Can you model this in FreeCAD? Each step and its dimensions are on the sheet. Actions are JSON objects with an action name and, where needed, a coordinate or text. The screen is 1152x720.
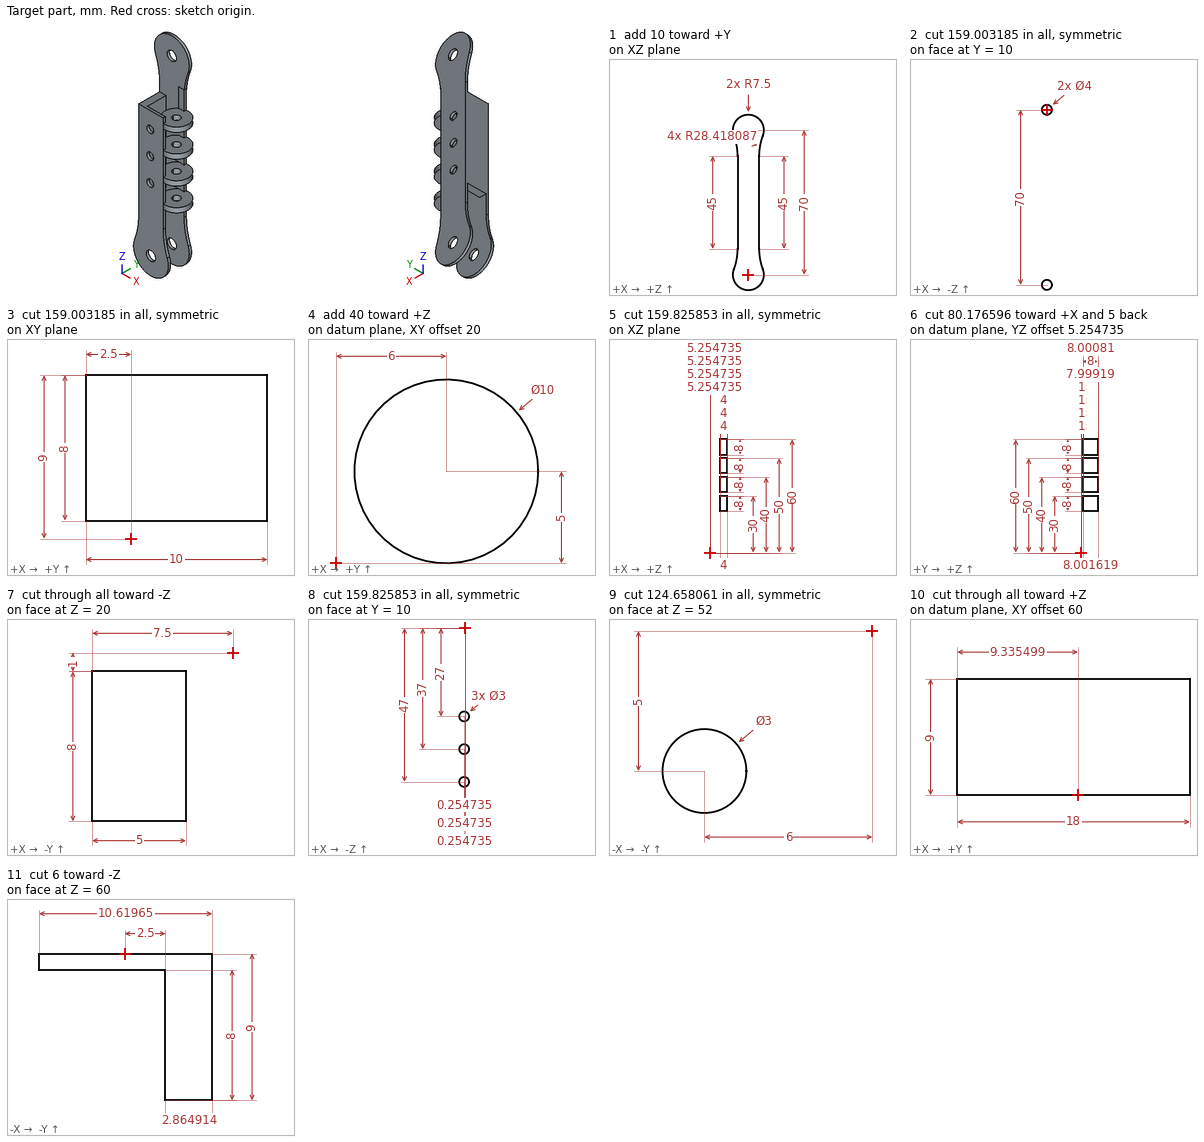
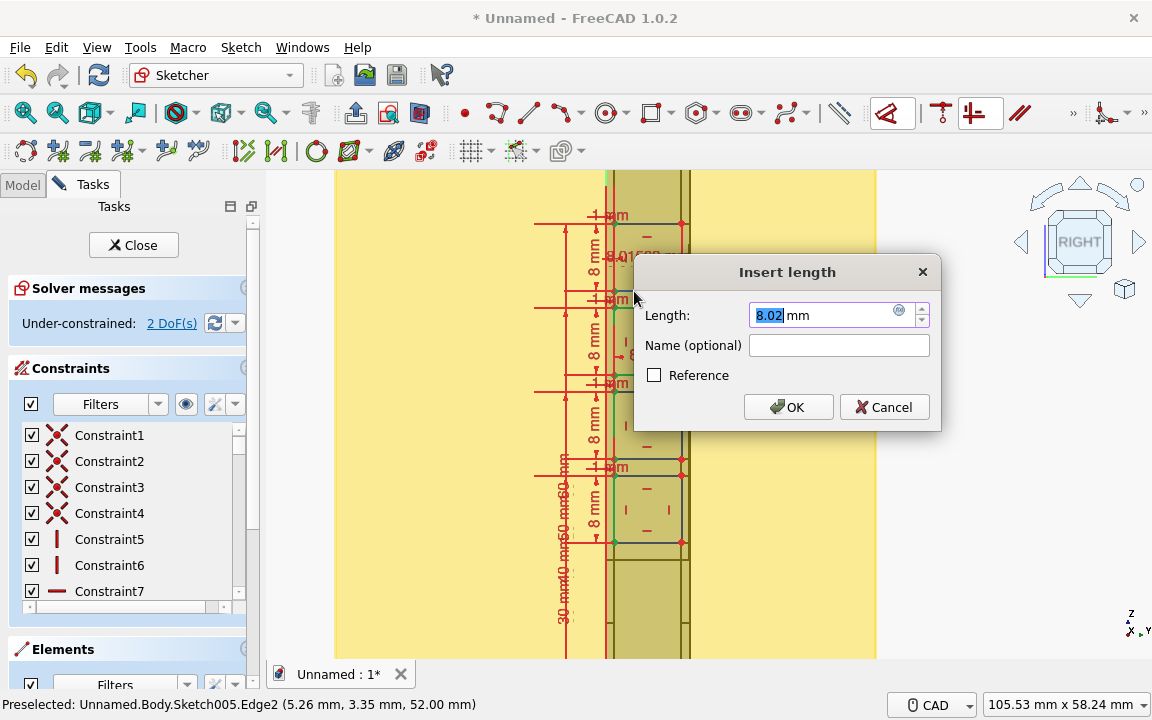
{"action": "type", "text": "7.99919"}
{"action": "key", "text": "Return"}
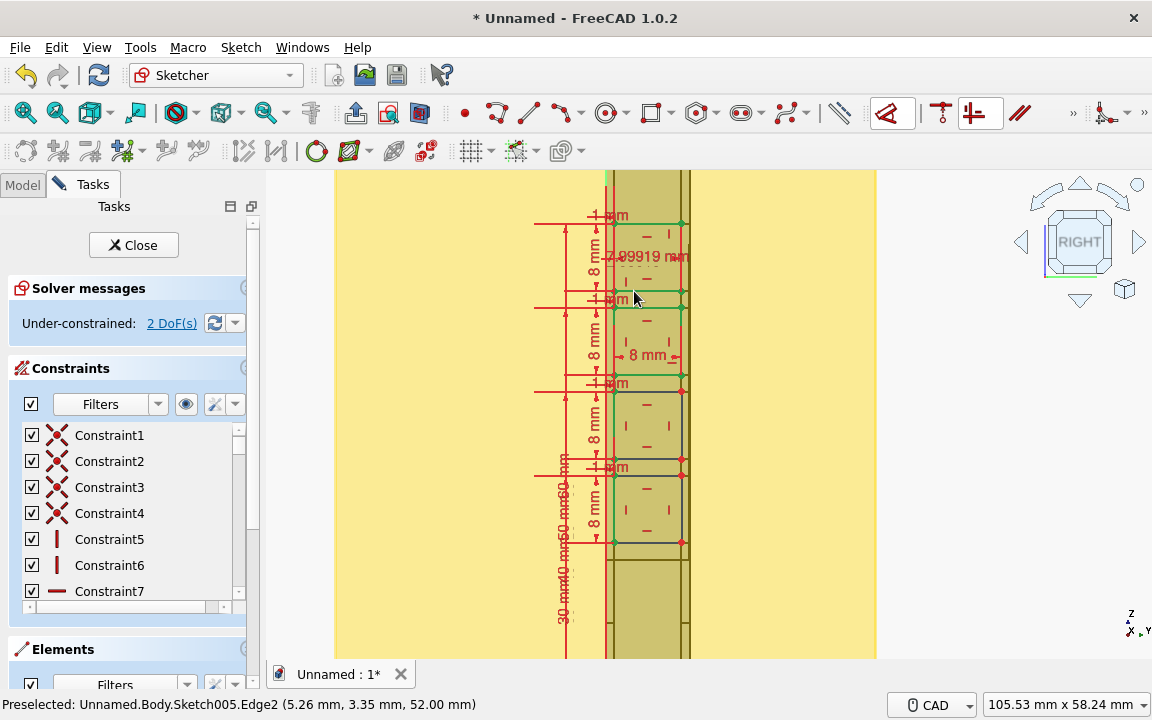
{"action": "left_click", "coordinate": [634, 459]}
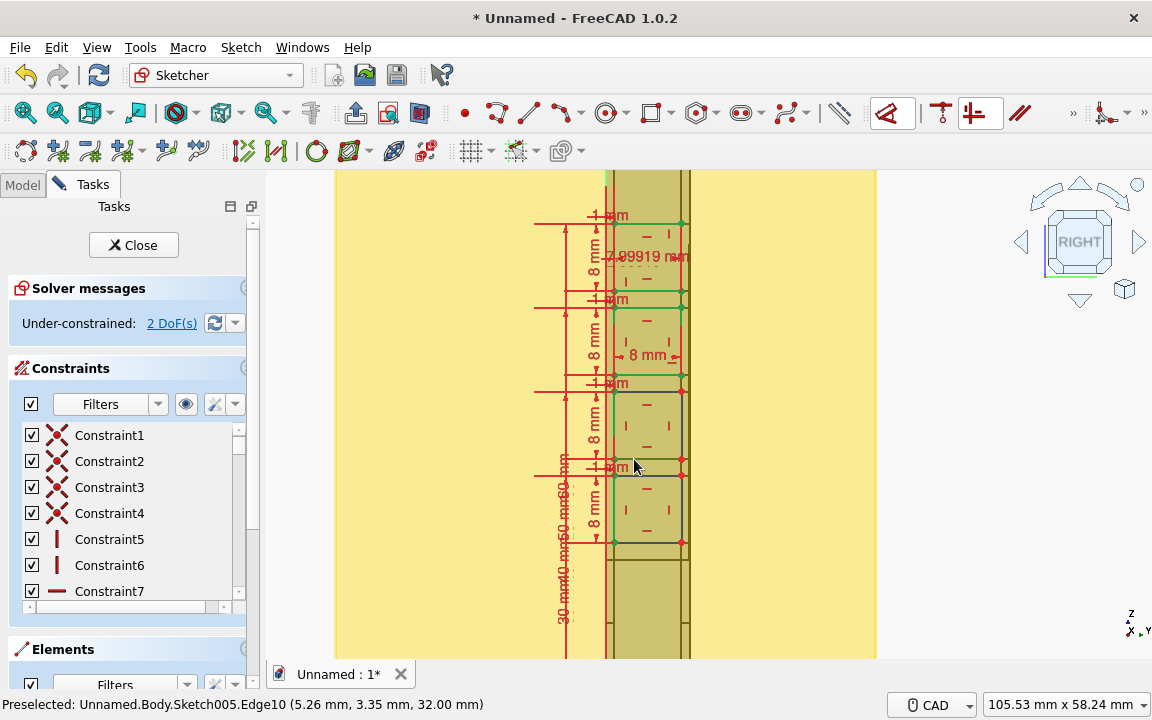
{"action": "key", "text": "l"}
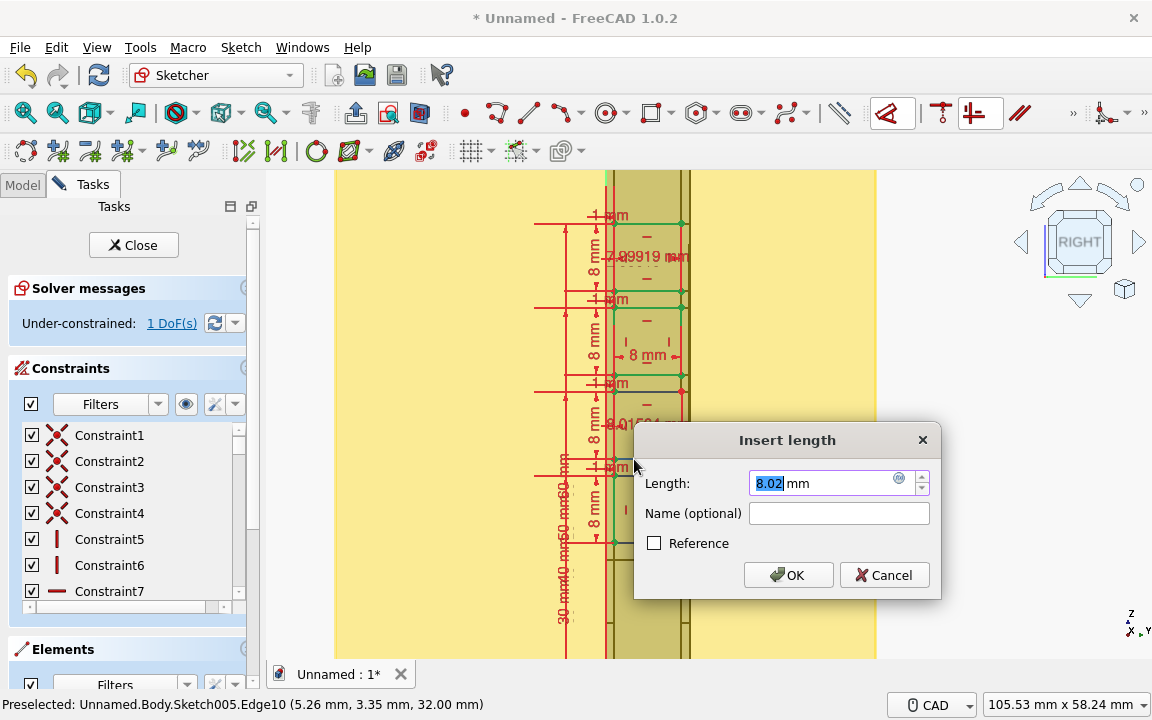
{"action": "type", "text": "8.00081"}
{"action": "key", "text": "Return"}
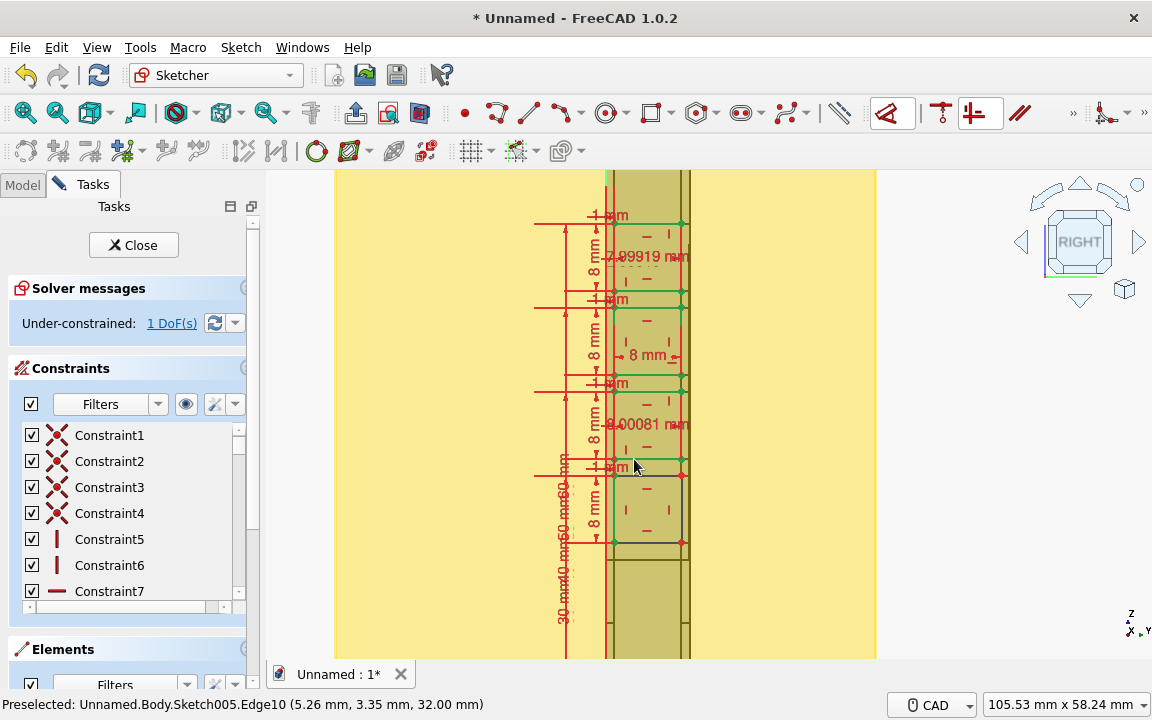
{"action": "left_click", "coordinate": [634, 543]}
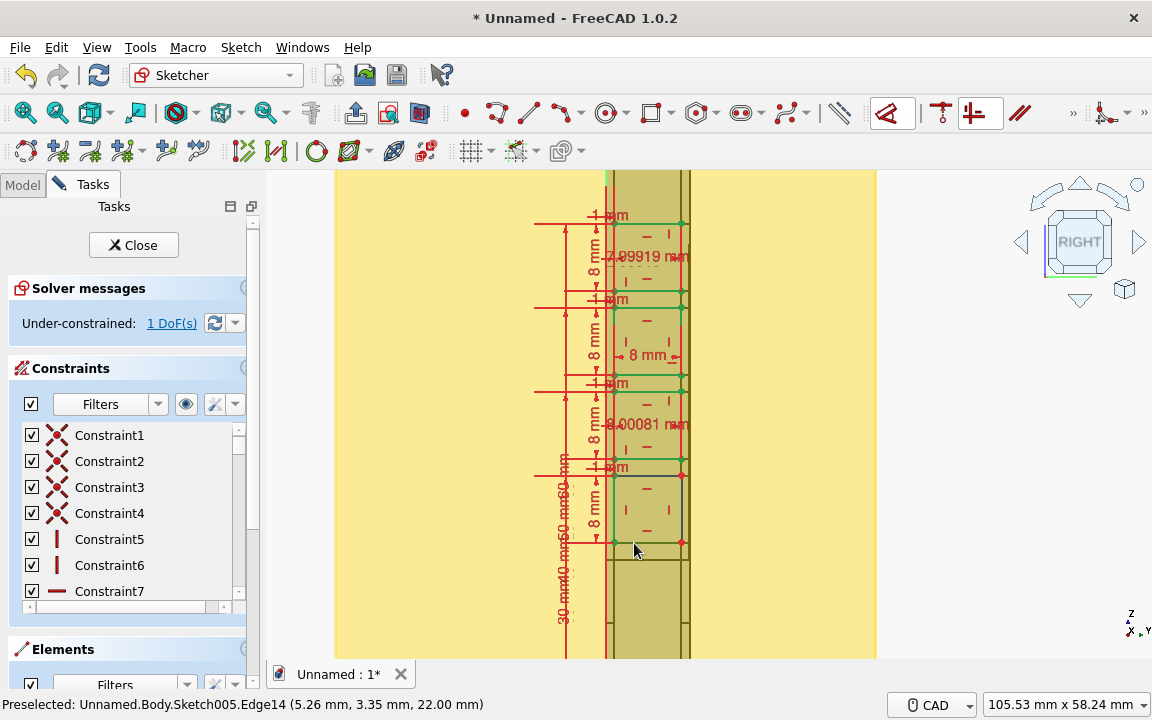
{"action": "left_click", "coordinate": [910, 114]}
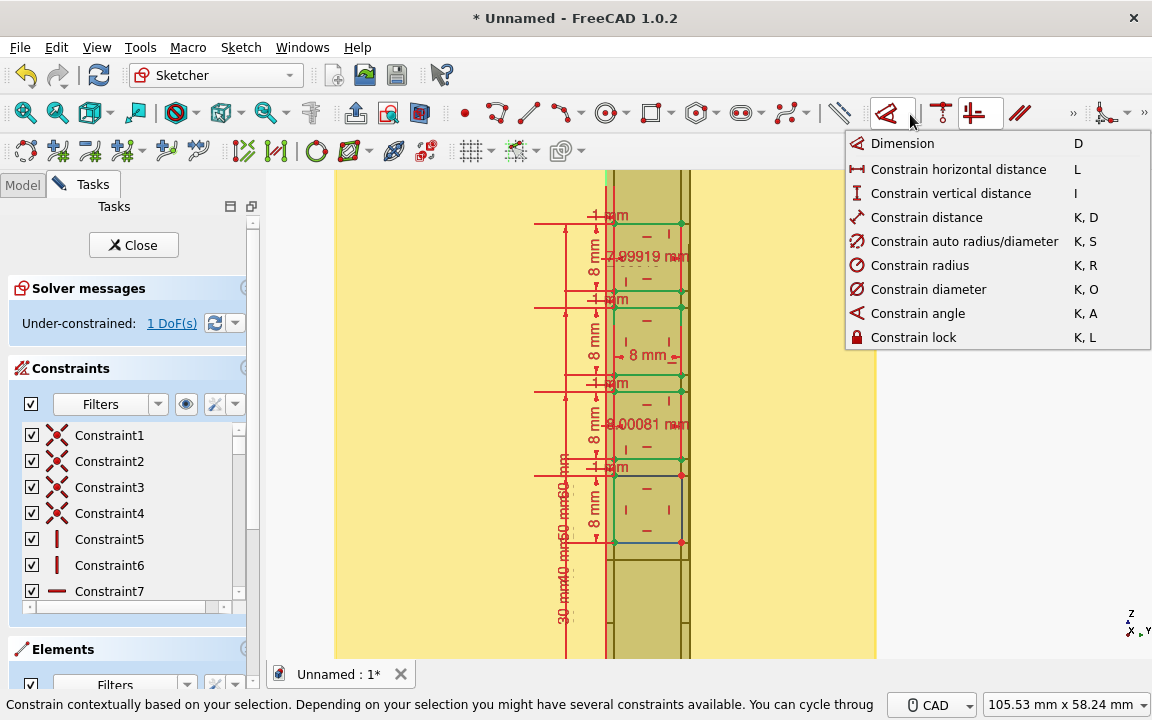
{"action": "left_click", "coordinate": [998, 169]}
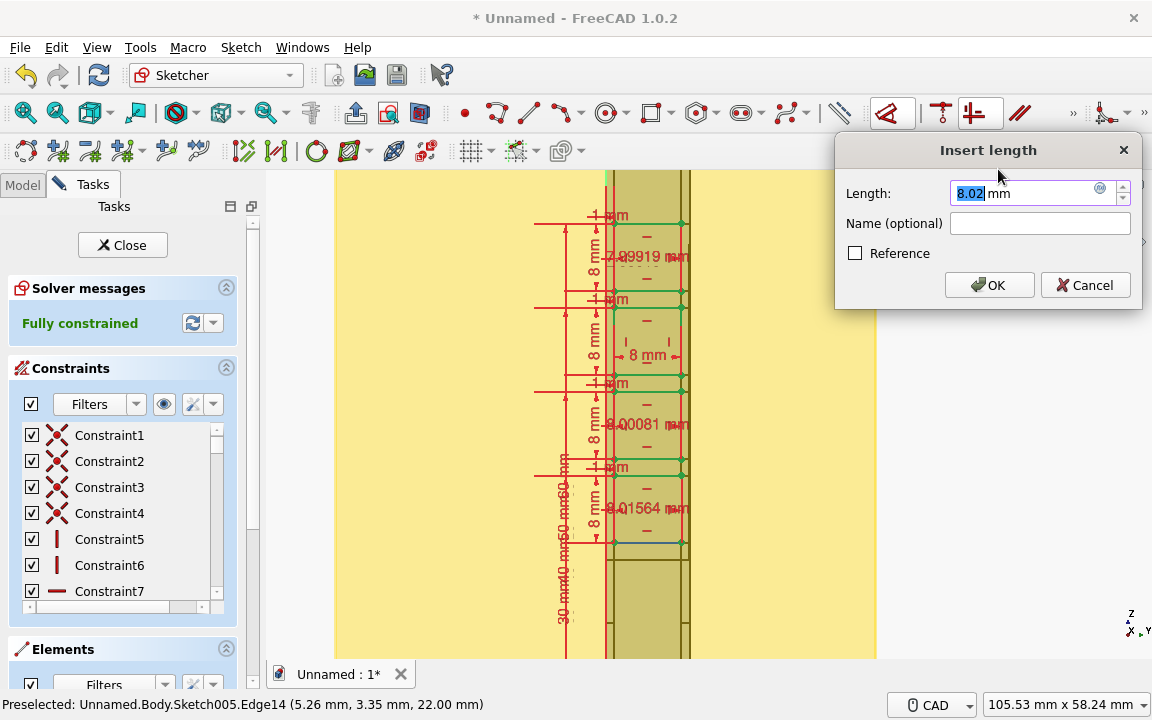
{"action": "type", "text": "8.001619"}
{"action": "key", "text": "Return"}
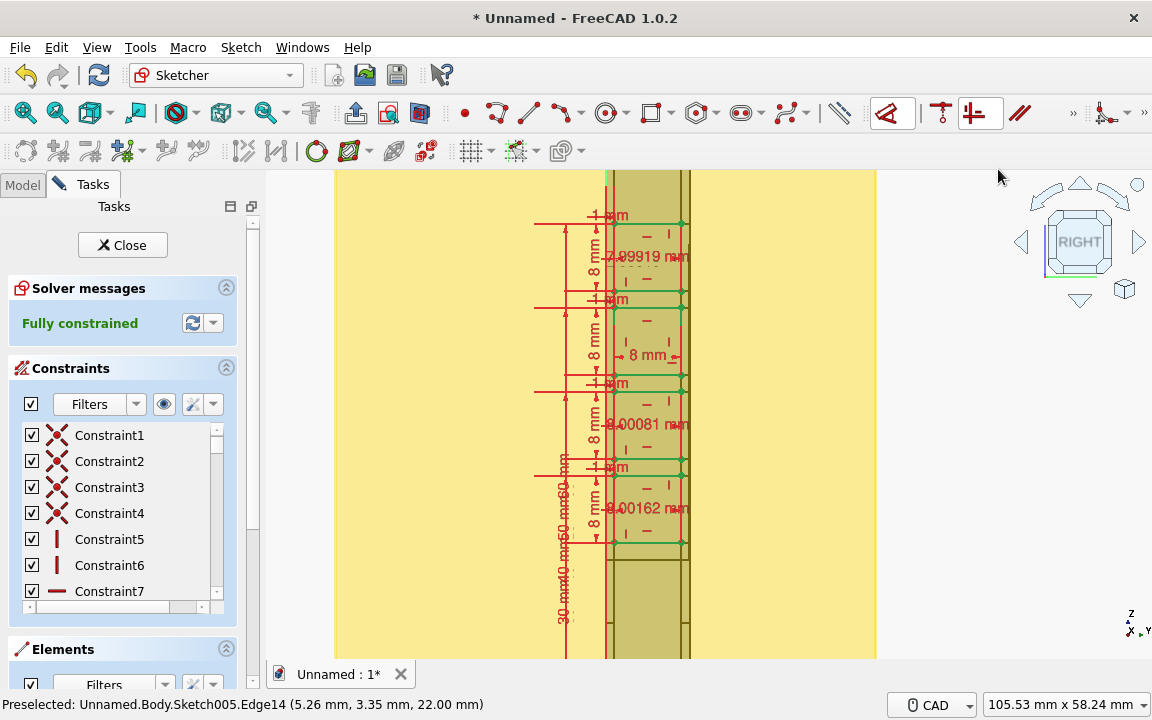
{"action": "left_click", "coordinate": [123, 245]}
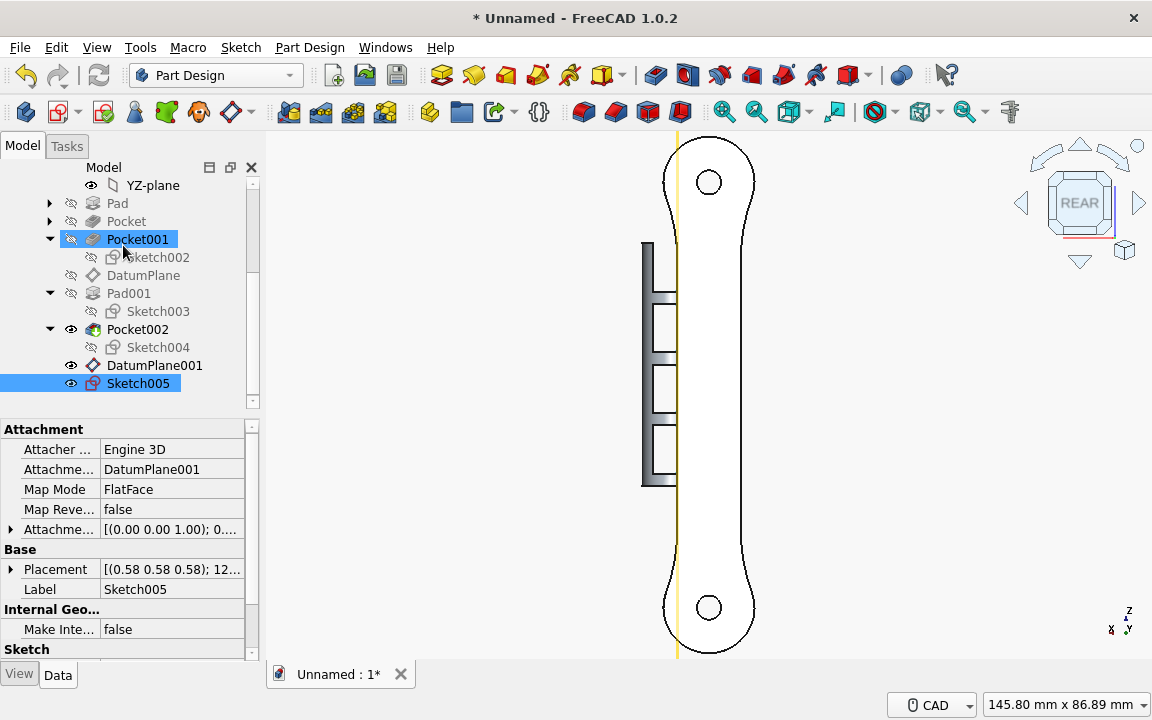
{"action": "left_click", "coordinate": [656, 76]}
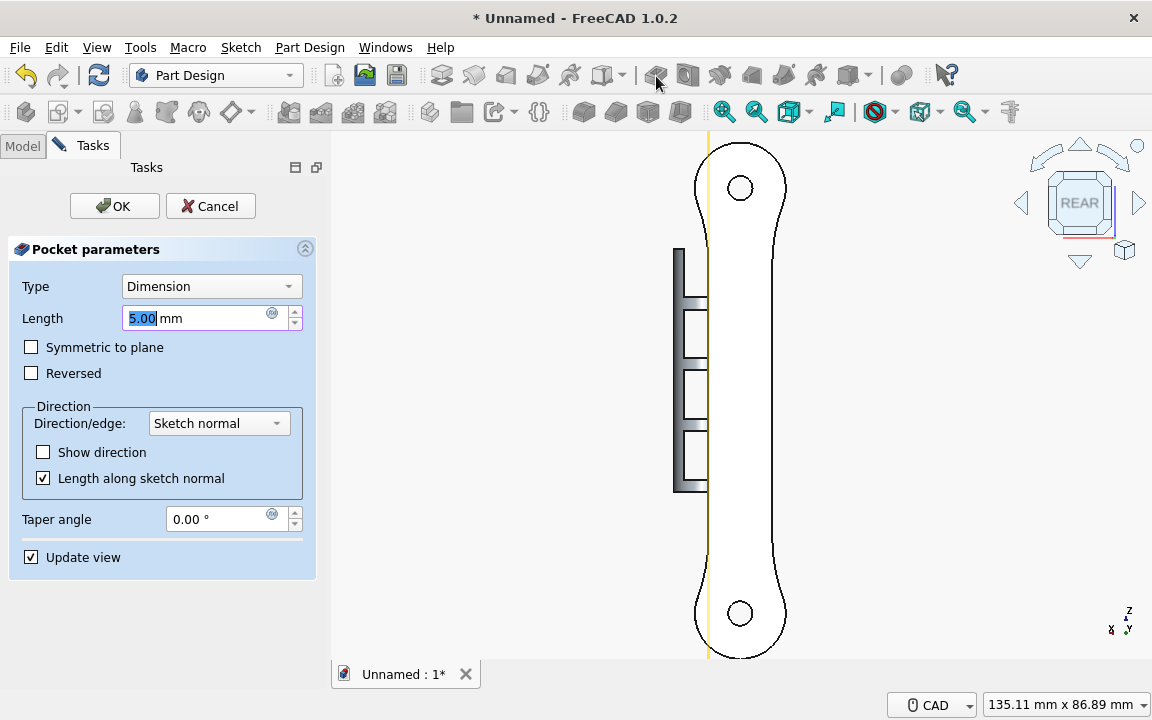
{"action": "left_click", "coordinate": [212, 286]}